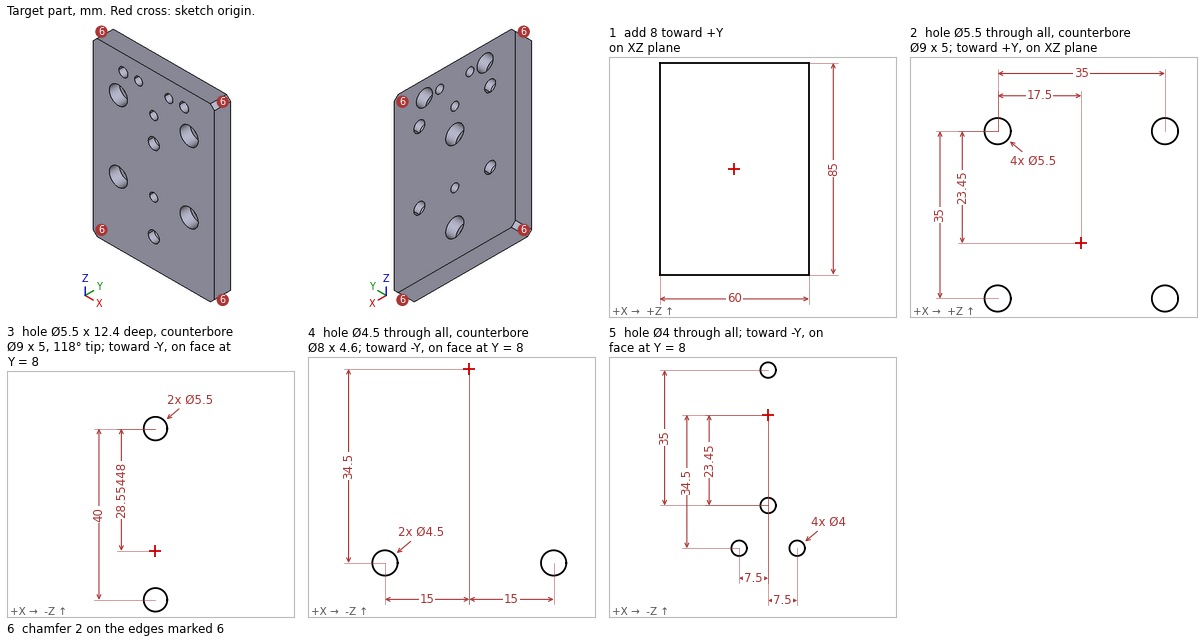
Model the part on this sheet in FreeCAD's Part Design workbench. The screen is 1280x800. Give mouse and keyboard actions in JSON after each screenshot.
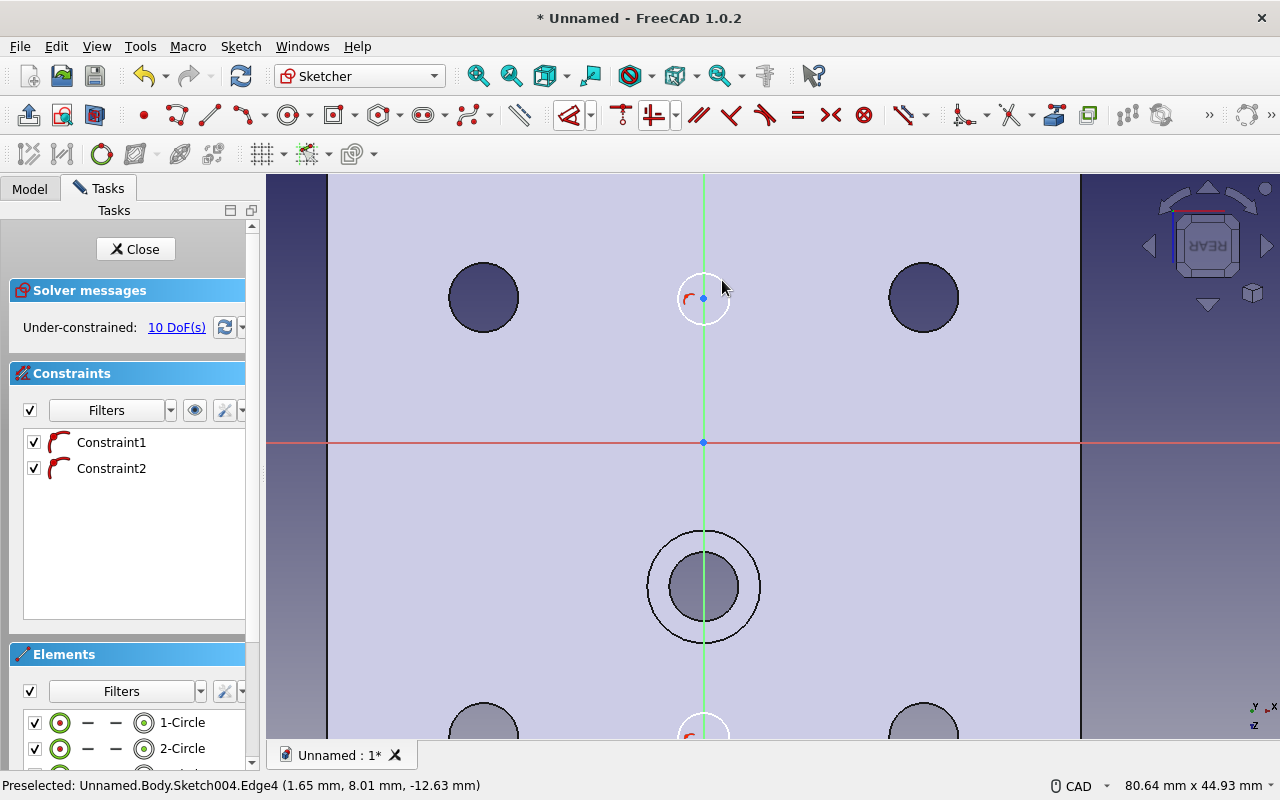
{"action": "scroll", "coordinate": [705, 298], "scroll_direction": "down", "scroll_amount": 3}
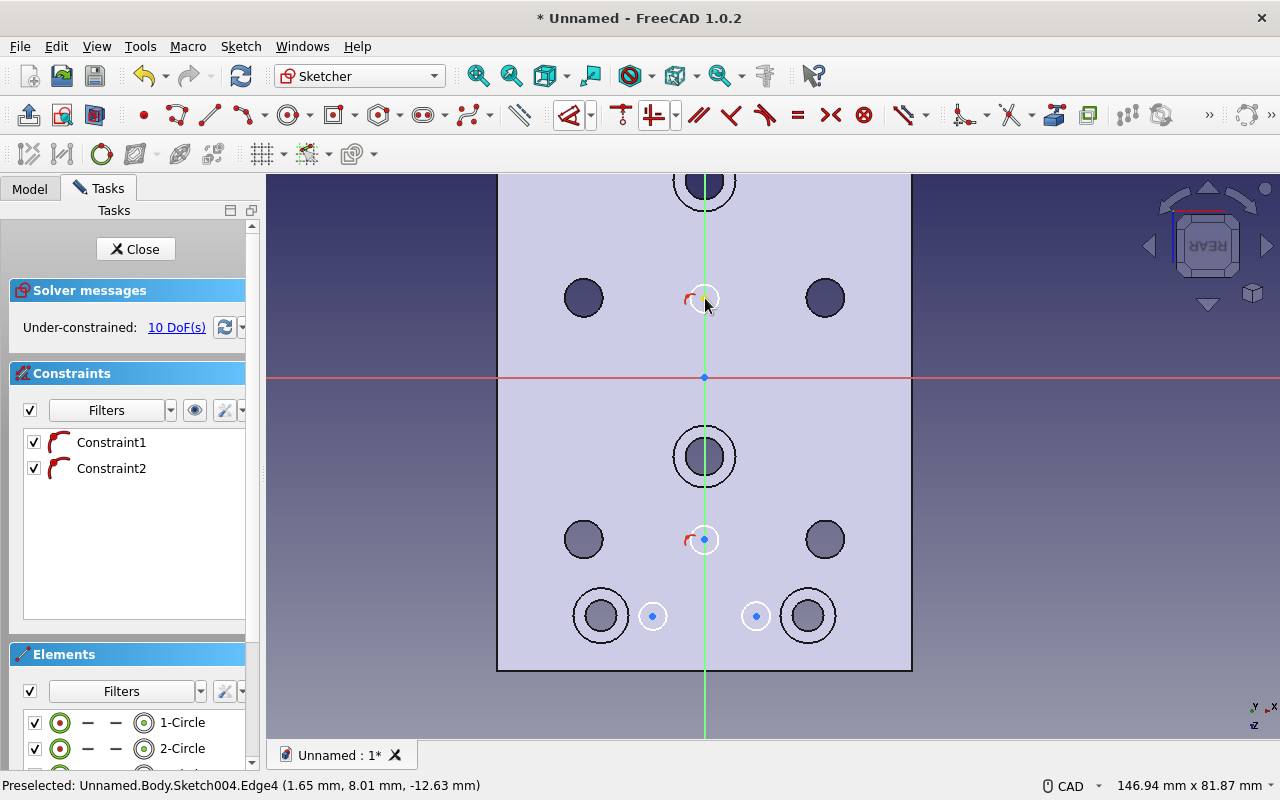
{"action": "left_click", "coordinate": [663, 607]}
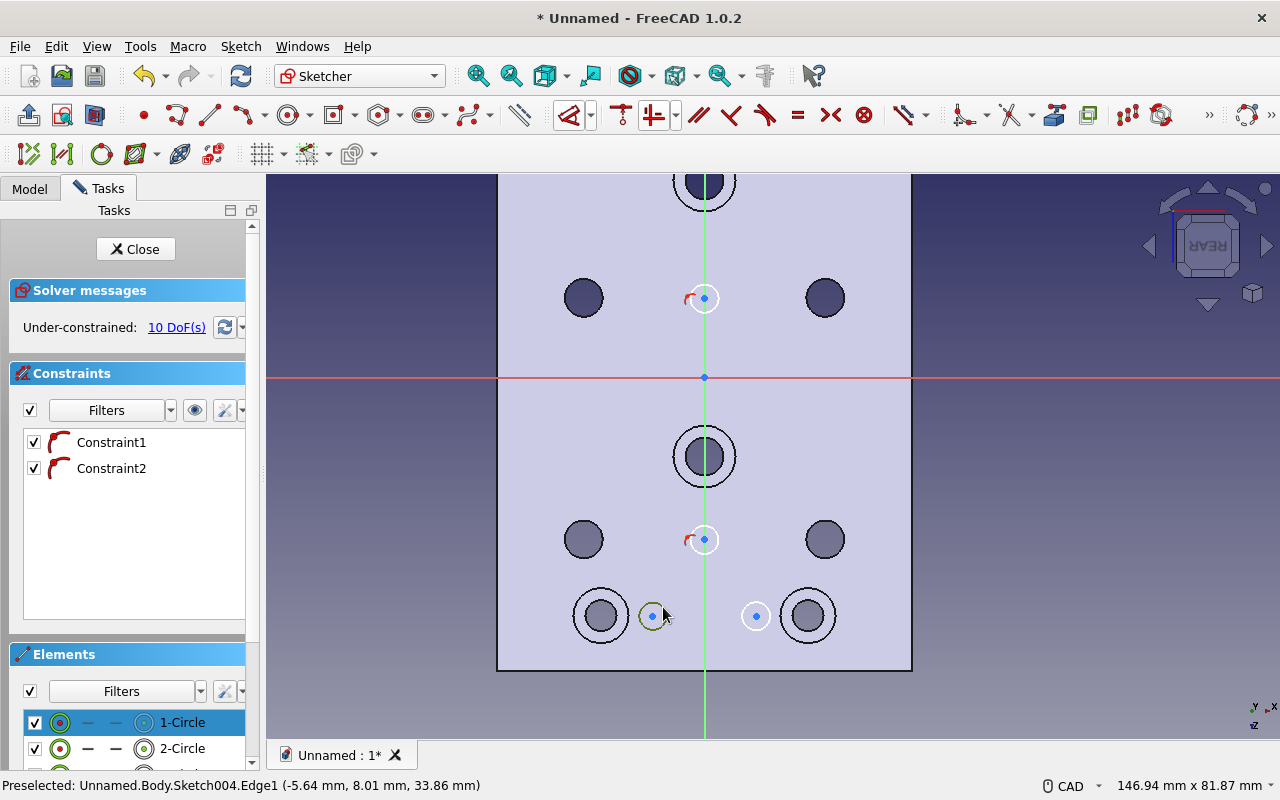
{"action": "left_click", "coordinate": [766, 606]}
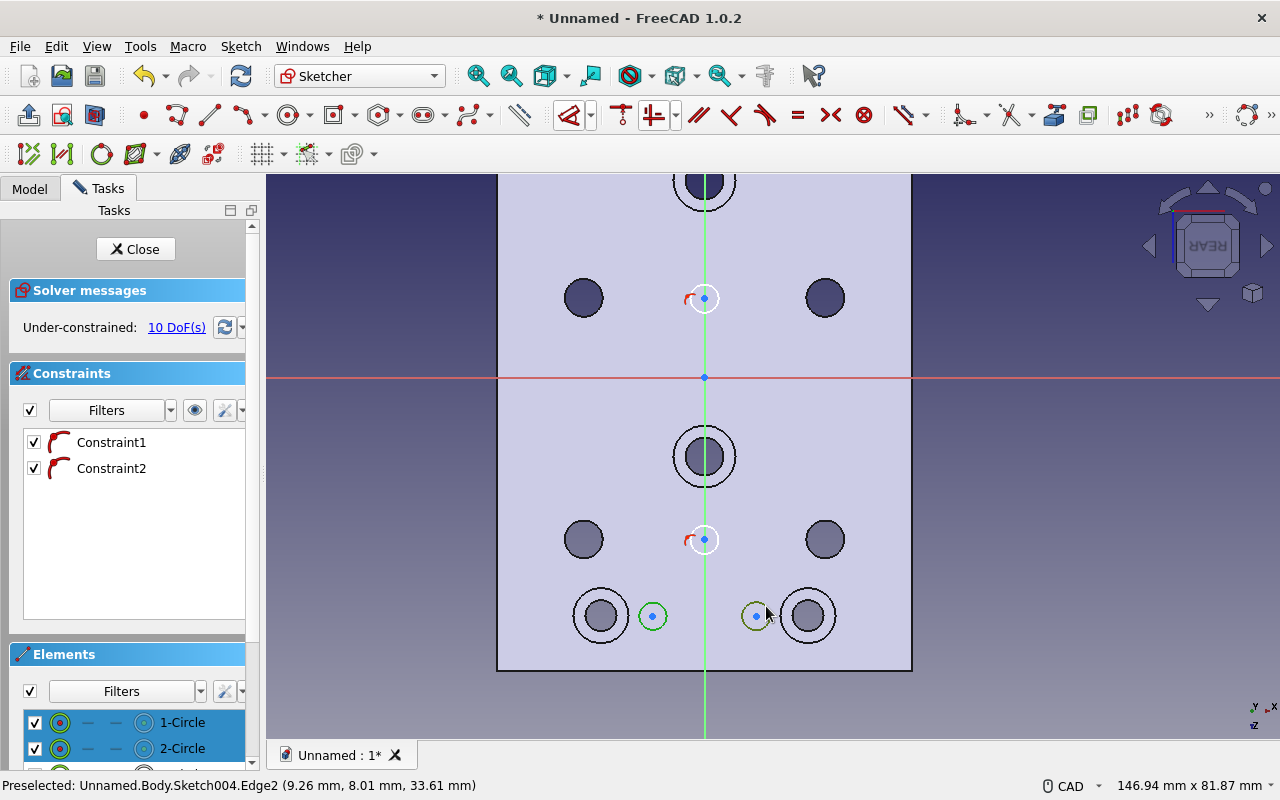
{"action": "scroll", "coordinate": [714, 530], "scroll_direction": "up", "scroll_amount": 2}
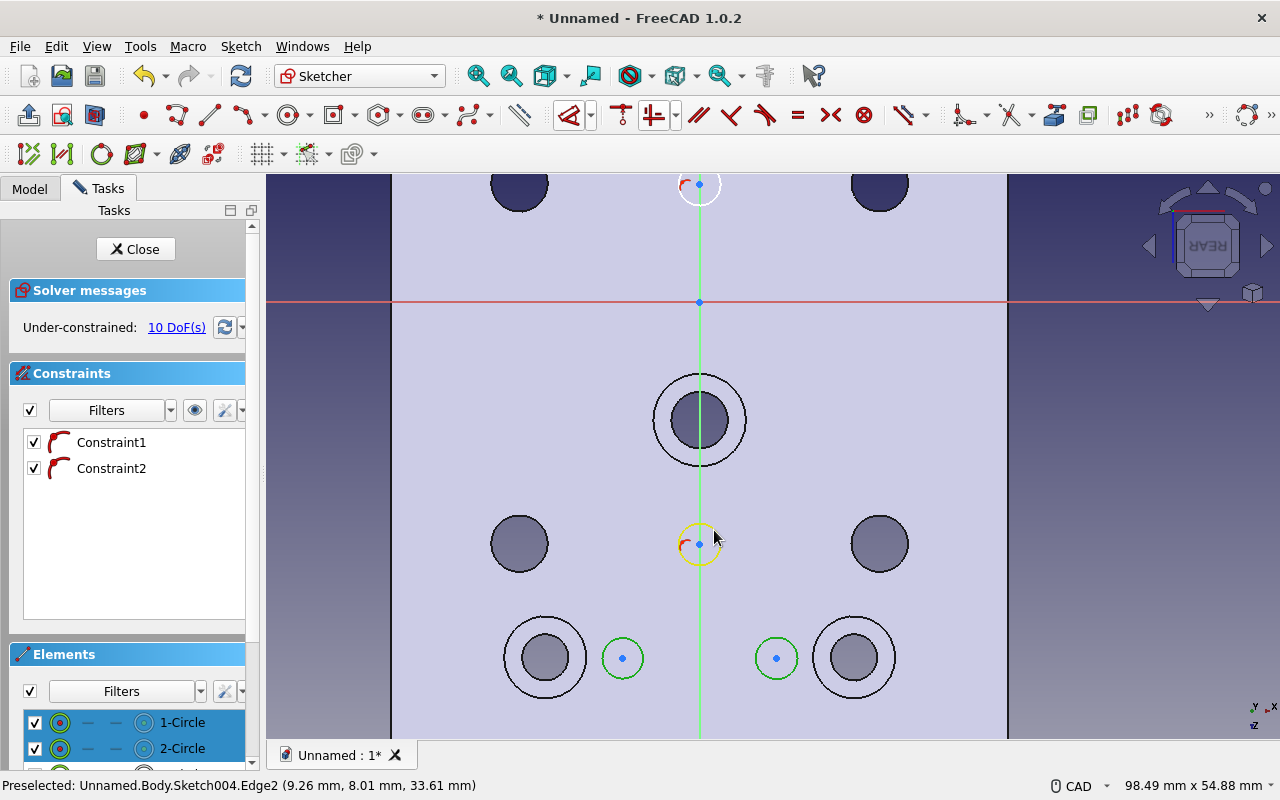
{"action": "left_click", "coordinate": [714, 530]}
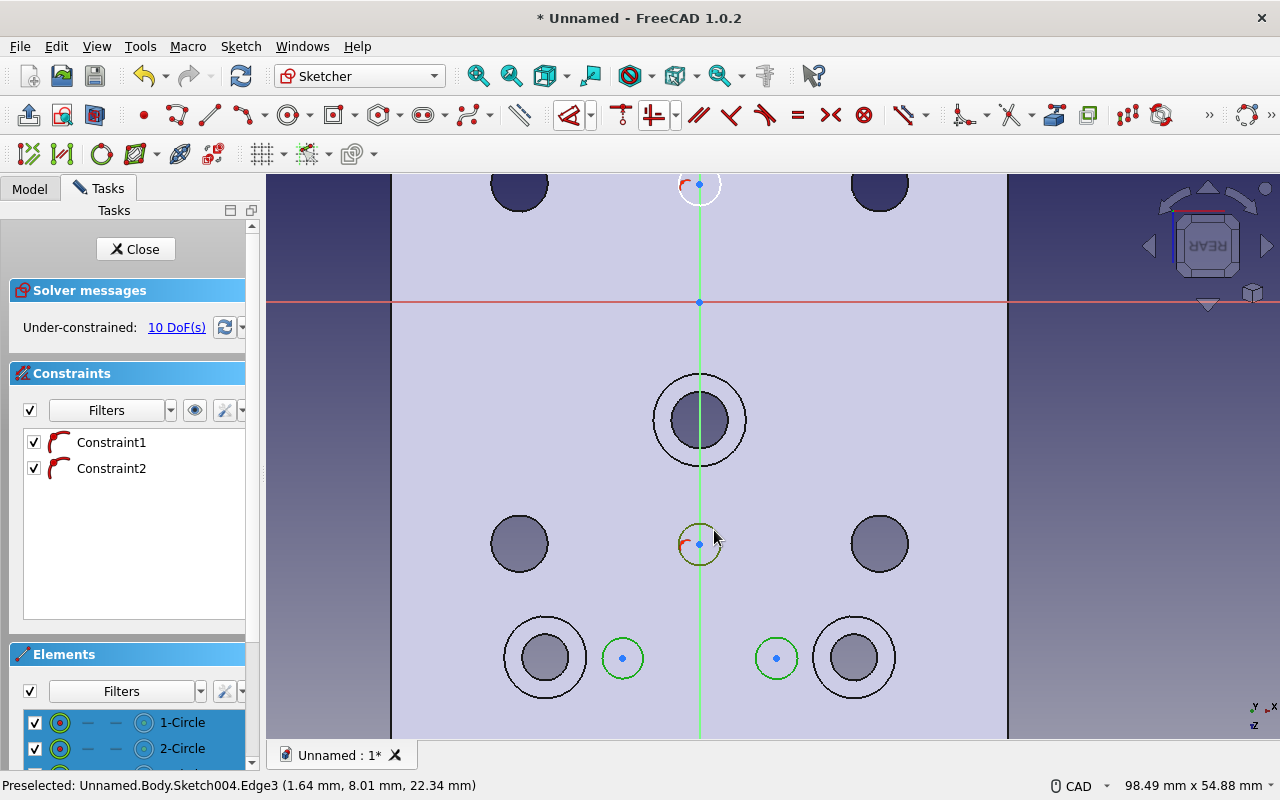
{"action": "left_click", "coordinate": [699, 206]}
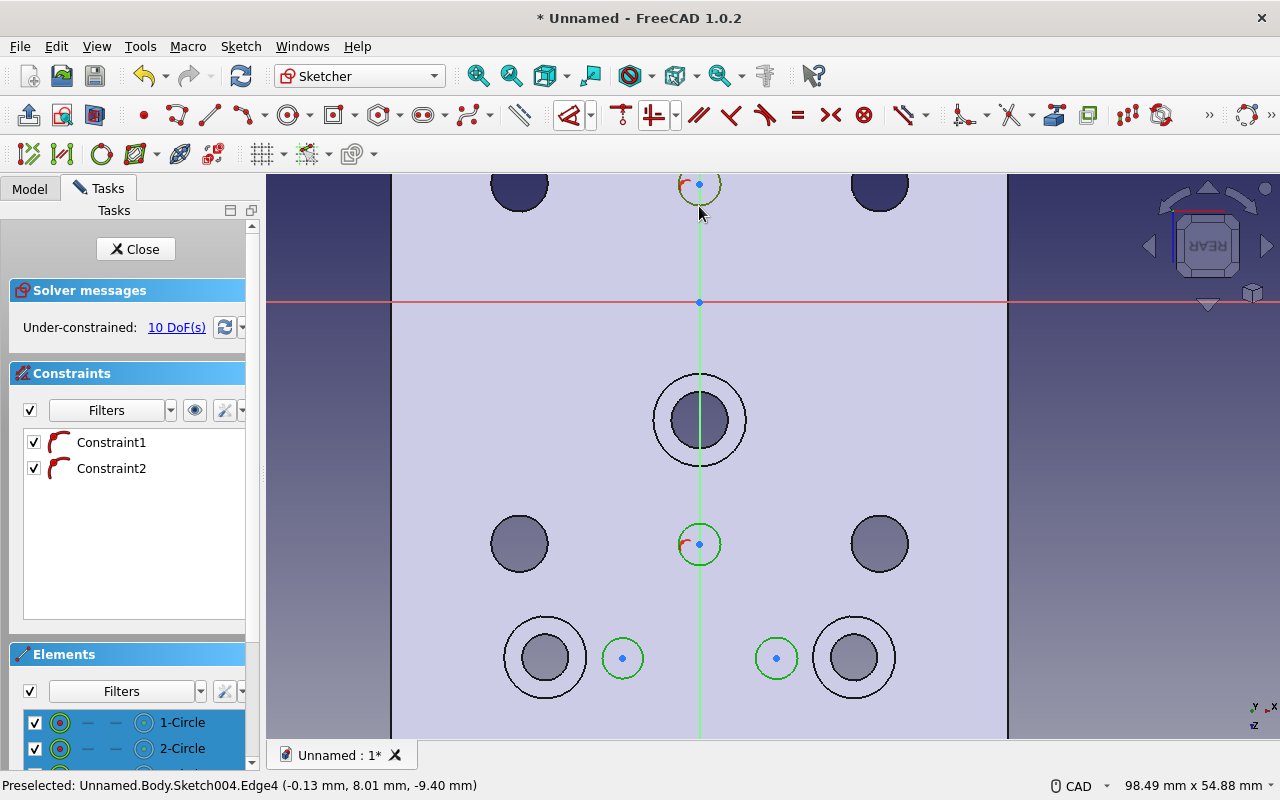
{"action": "left_click", "coordinate": [798, 116]}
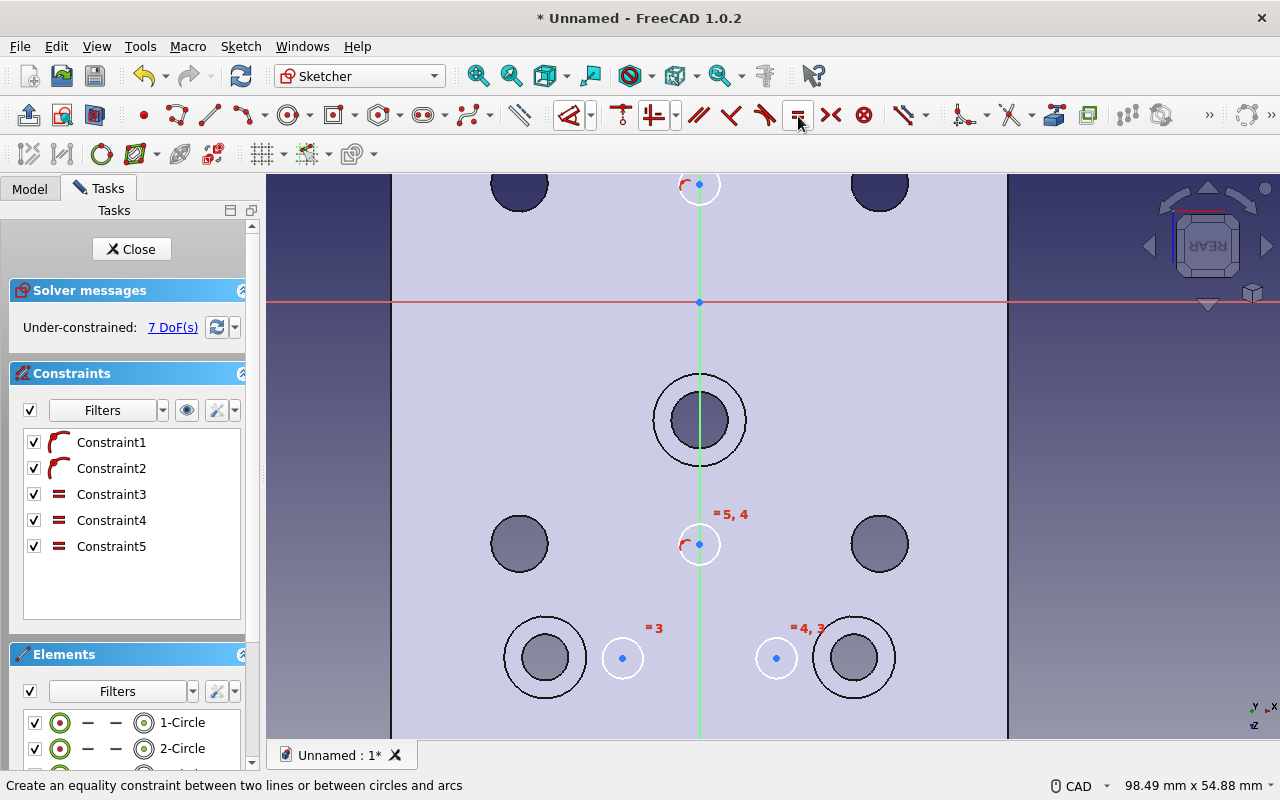
{"action": "left_click", "coordinate": [623, 658]}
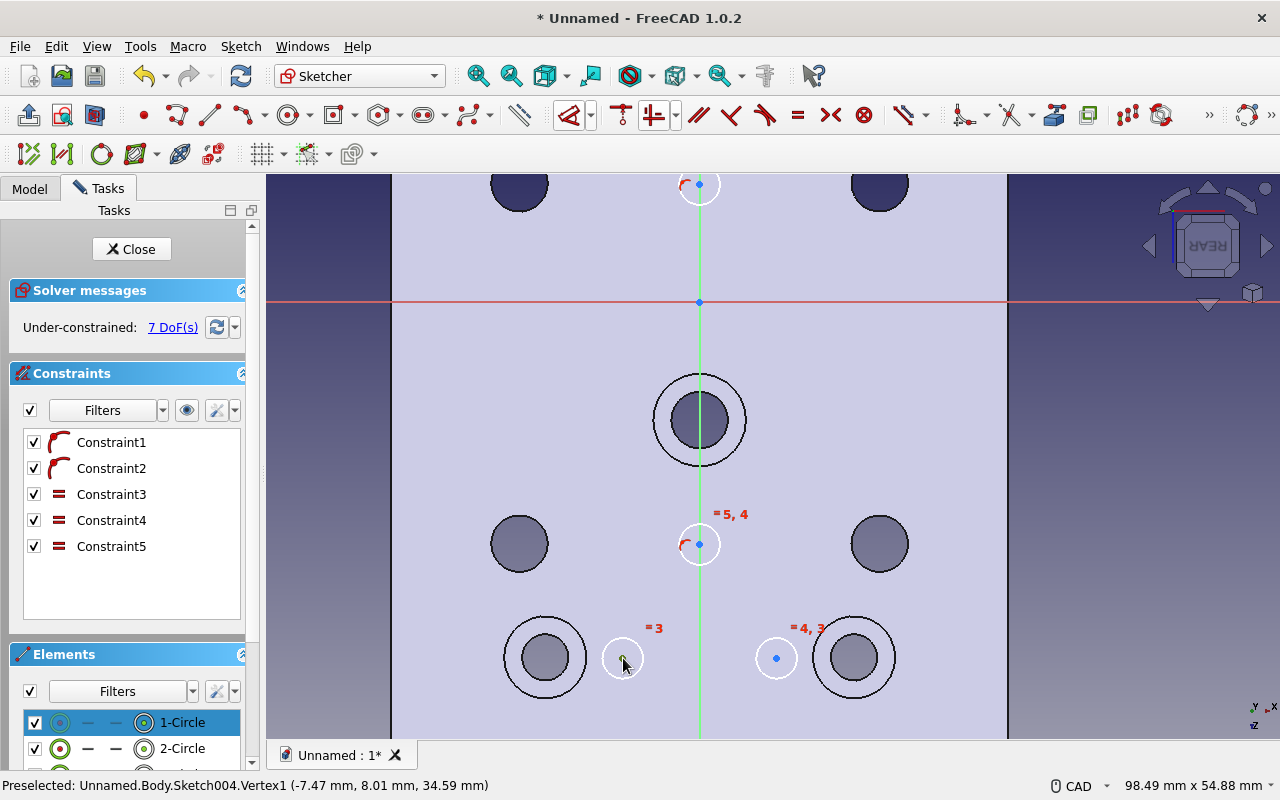
{"action": "left_click", "coordinate": [777, 658]}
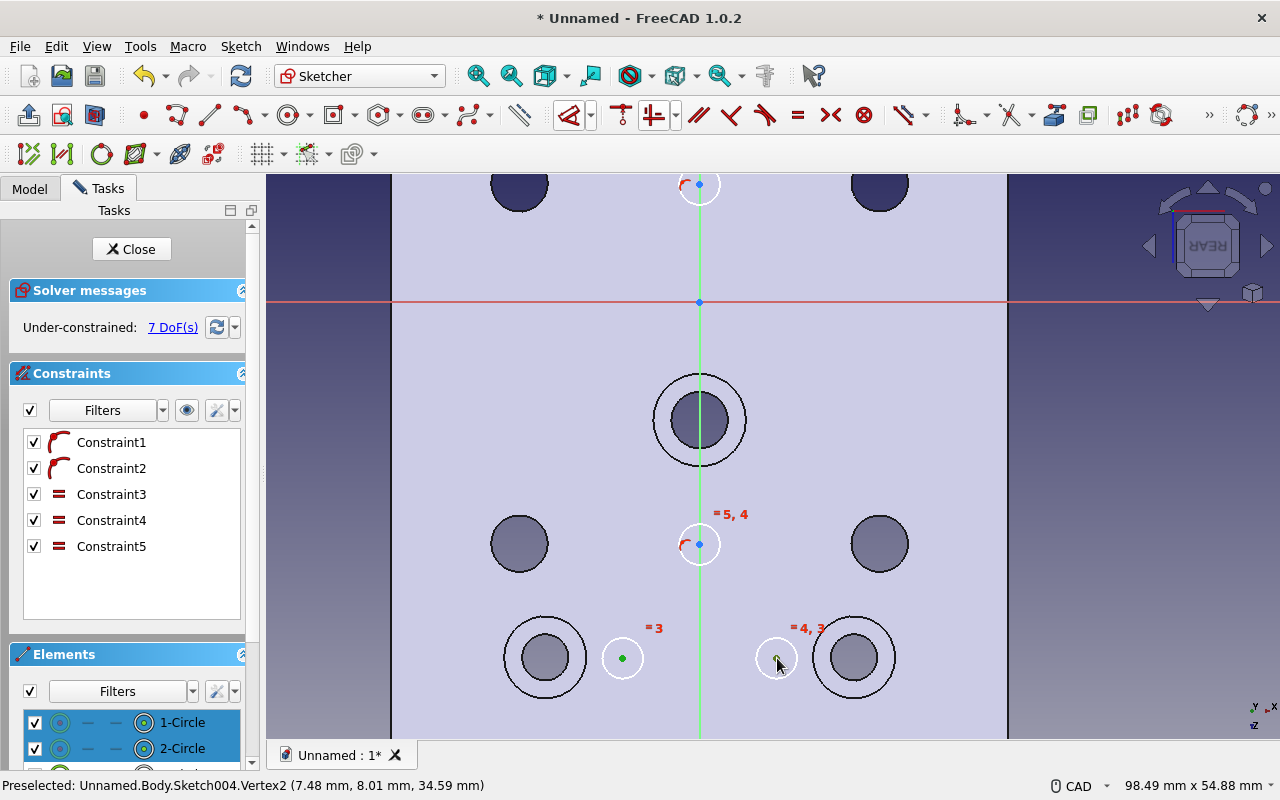
{"action": "key", "text": "h"}